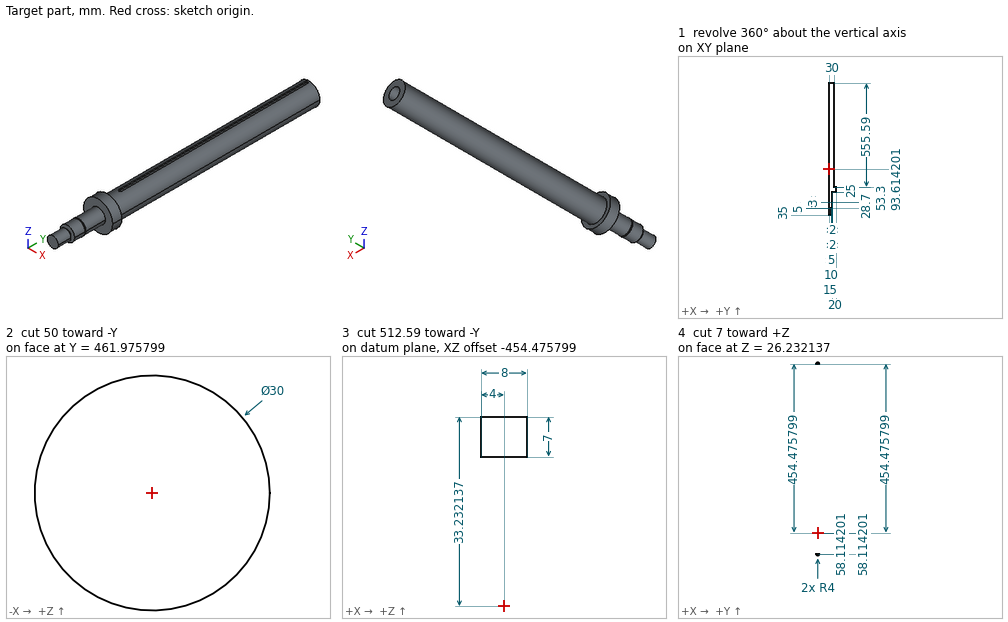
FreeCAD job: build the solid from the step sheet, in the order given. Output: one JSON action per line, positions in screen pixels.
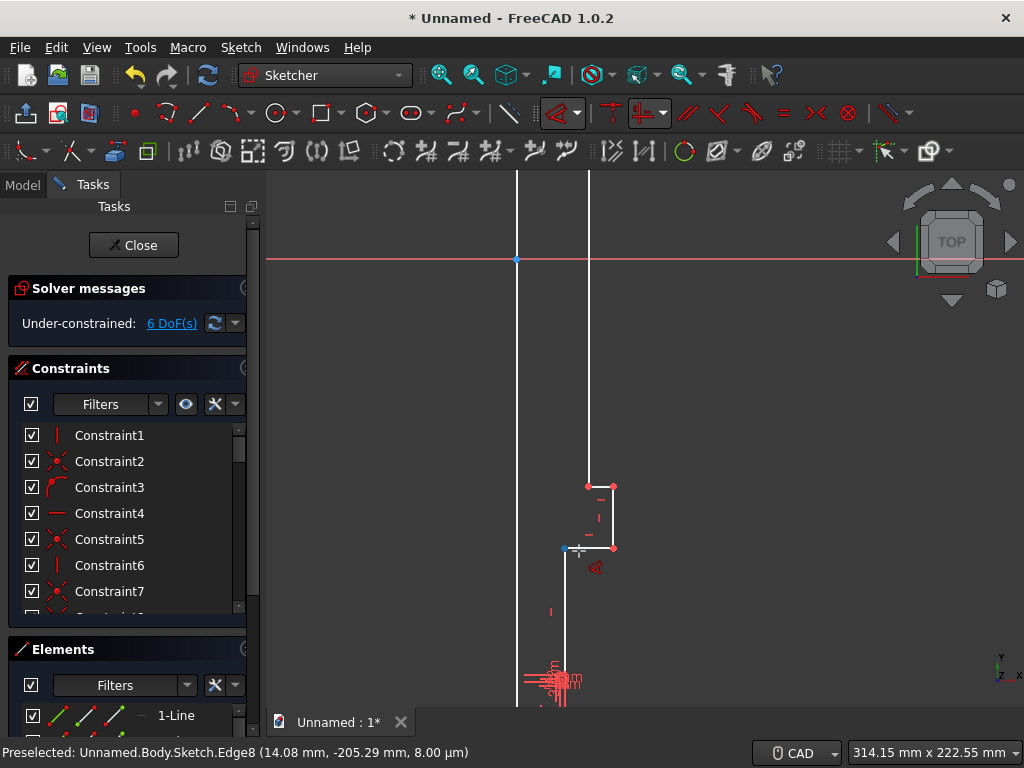
{"action": "left_click", "coordinate": [579, 548]}
{"action": "left_click", "coordinate": [589, 582]}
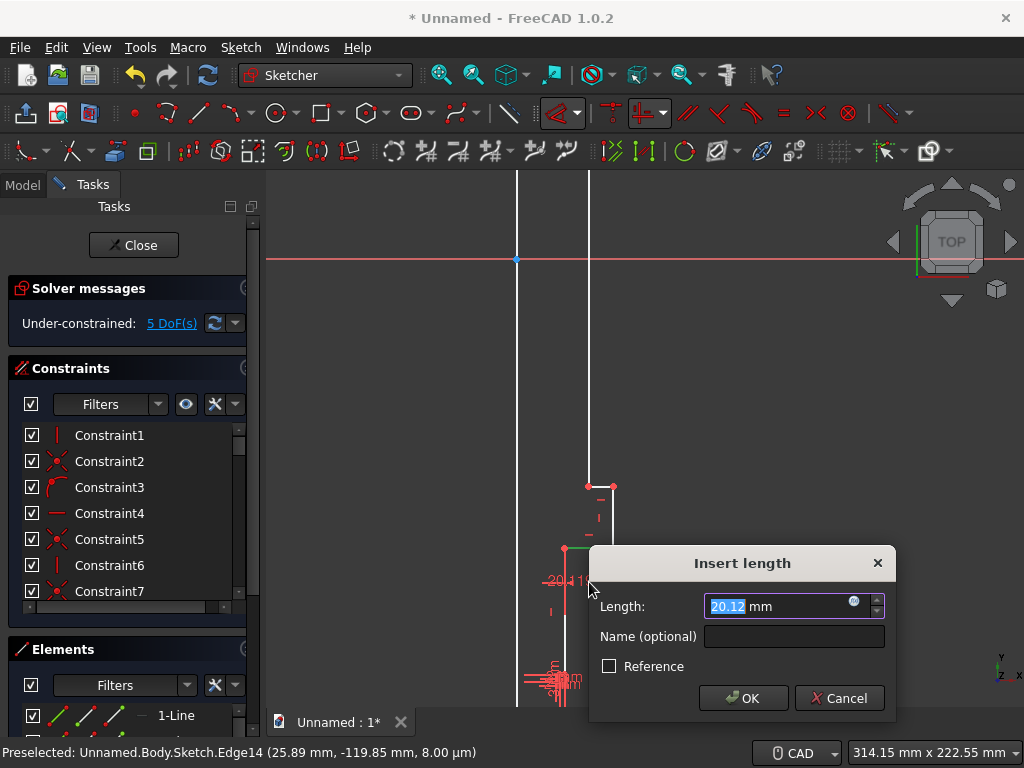
{"action": "type", "text": "20"}
{"action": "key", "text": "Return"}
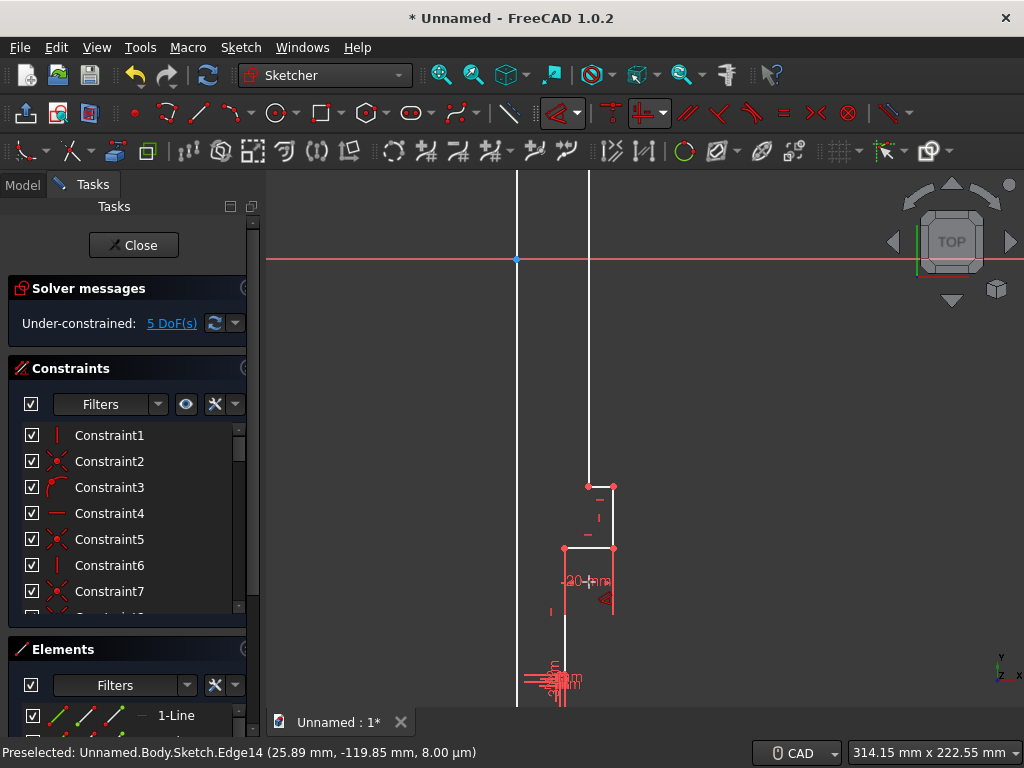
{"action": "left_click", "coordinate": [613, 530]}
{"action": "left_click", "coordinate": [647, 517]}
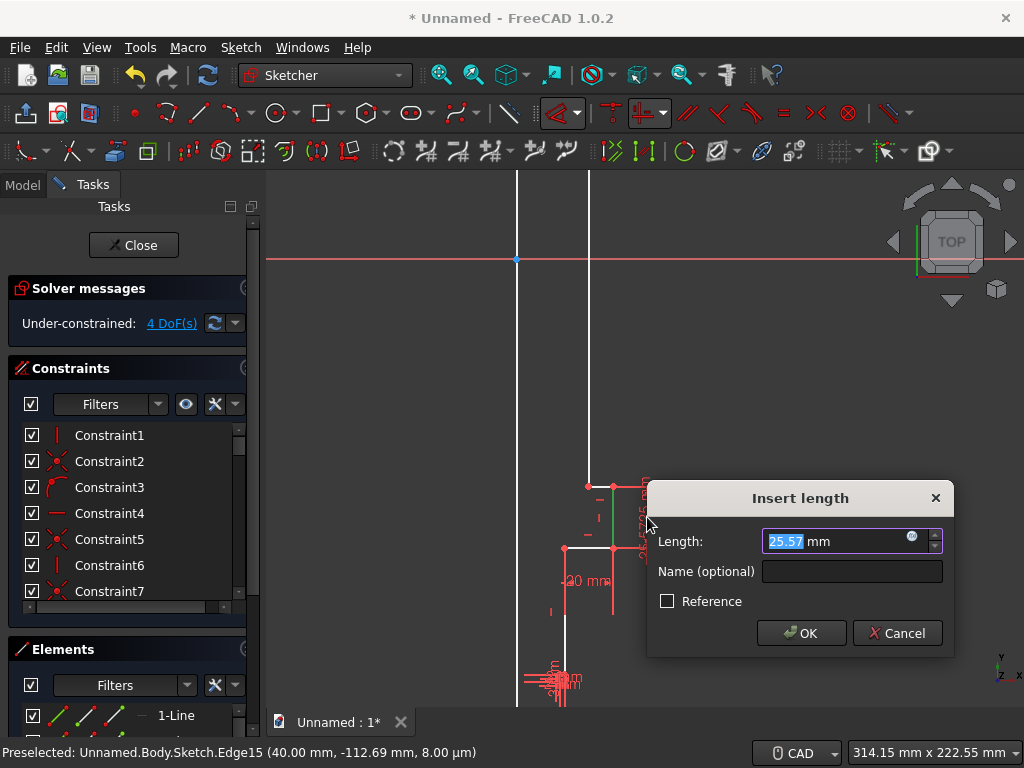
{"action": "type", "text": "25"}
{"action": "key", "text": "Return"}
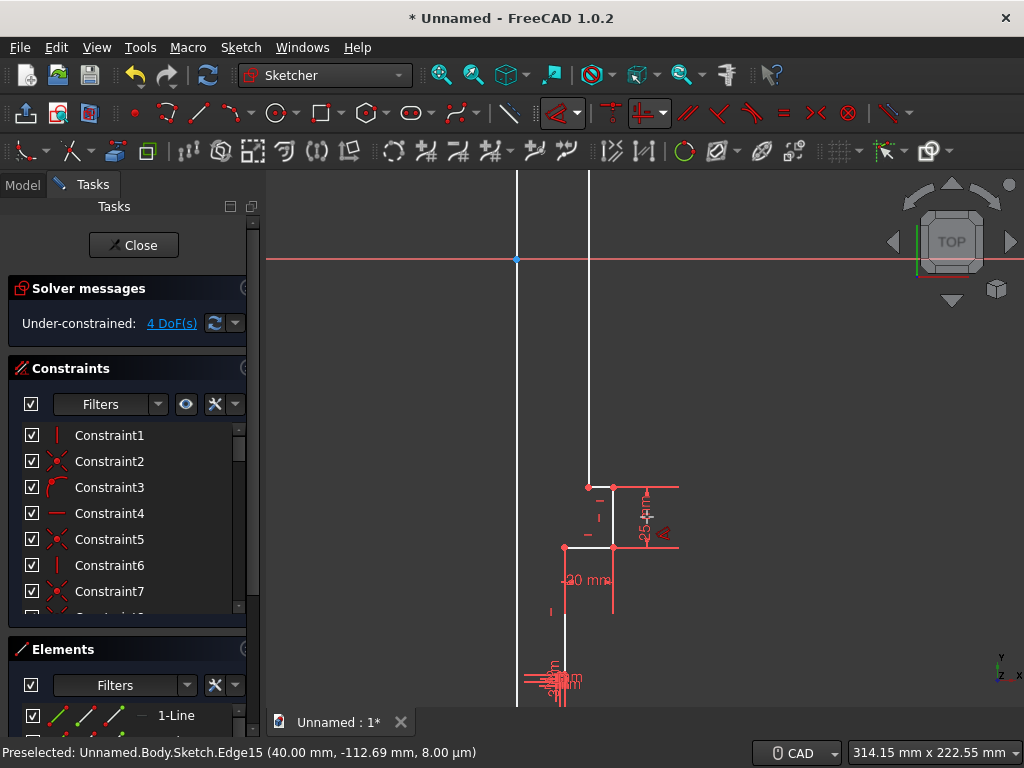
{"action": "scroll", "coordinate": [579, 551], "scroll_direction": "down", "scroll_amount": 8}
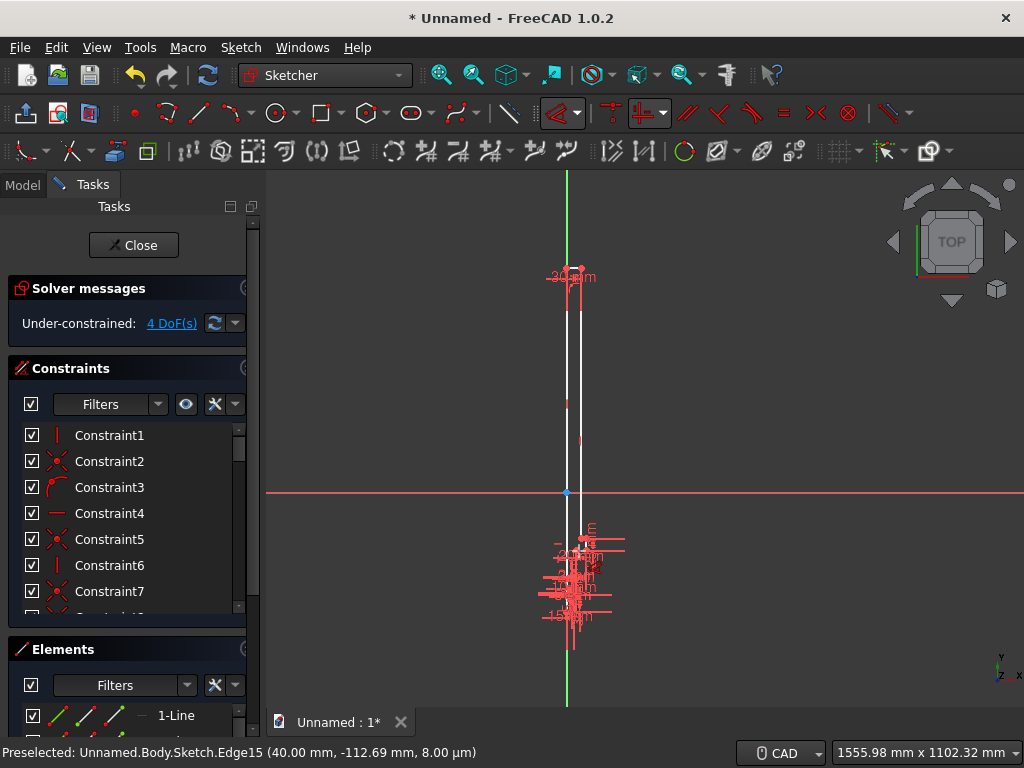
{"action": "scroll", "coordinate": [576, 588], "scroll_direction": "up", "scroll_amount": 6}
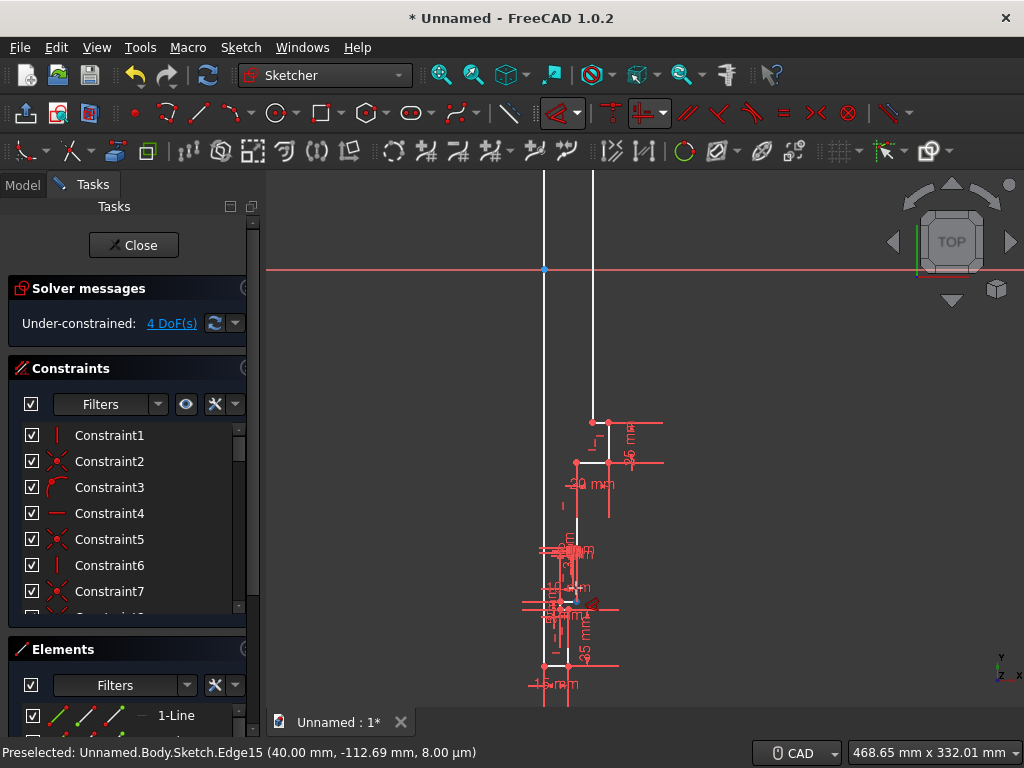
{"action": "left_click", "coordinate": [577, 587]}
{"action": "left_click", "coordinate": [659, 577]}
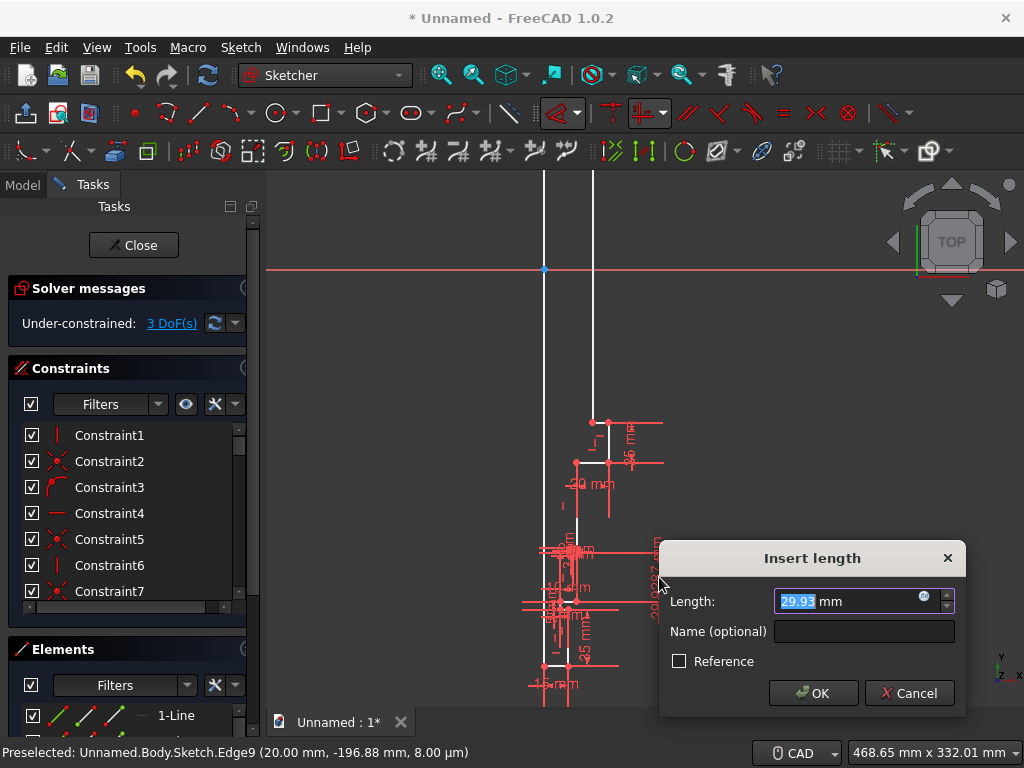
{"action": "type", "text": "28.7"}
{"action": "key", "text": "Return"}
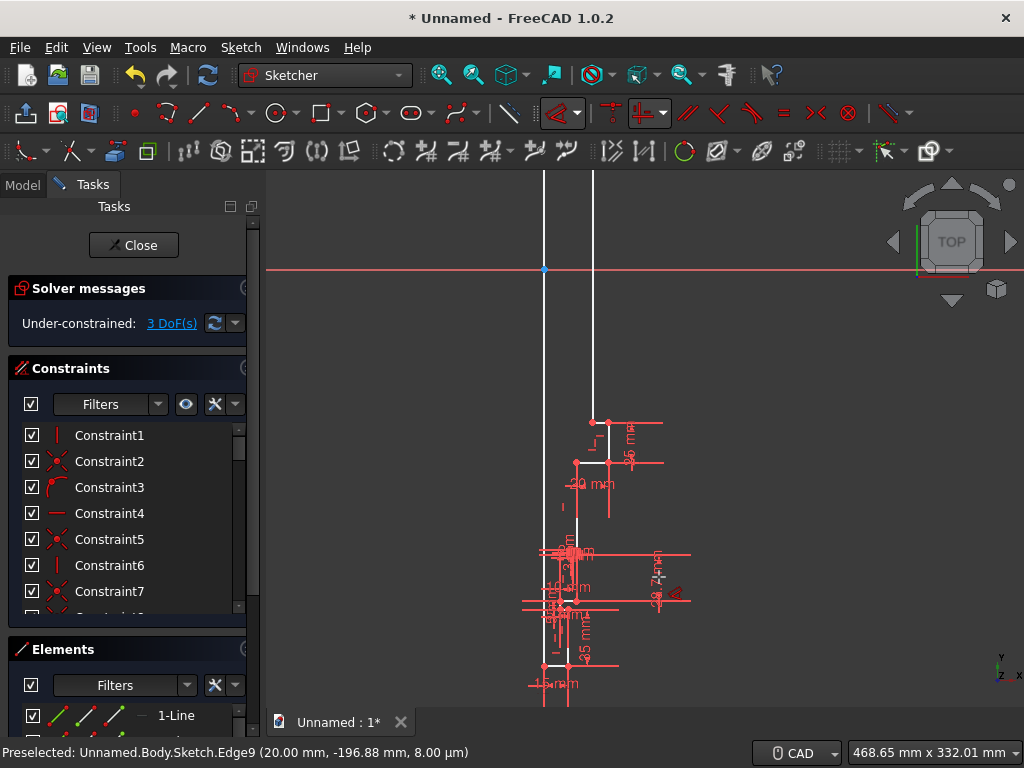
{"action": "left_click", "coordinate": [577, 524]}
{"action": "left_click", "coordinate": [611, 507]}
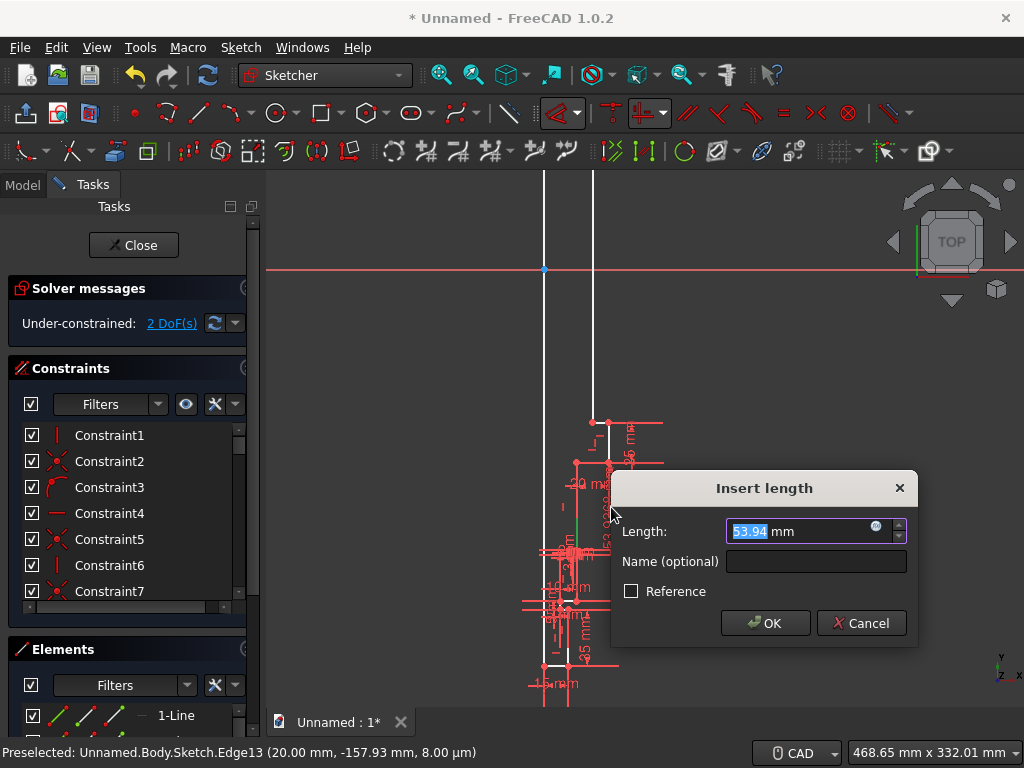
{"action": "type", "text": "53.3"}
{"action": "key", "text": "Return"}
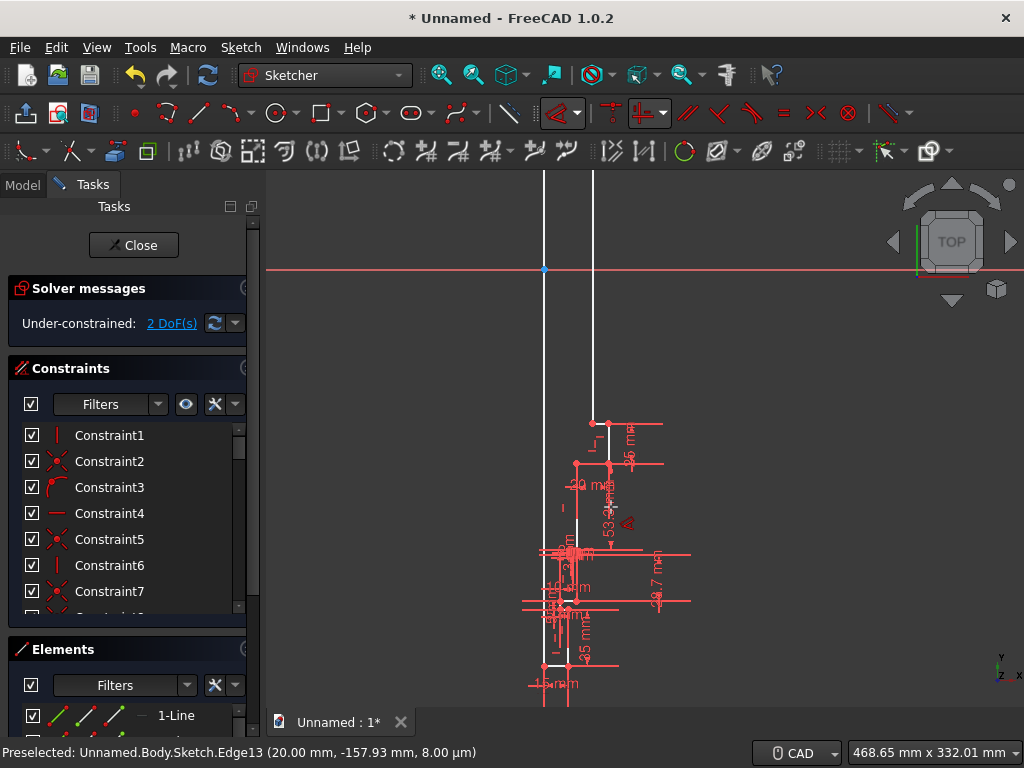
{"action": "left_click", "coordinate": [593, 244]}
{"action": "left_click", "coordinate": [627, 311]}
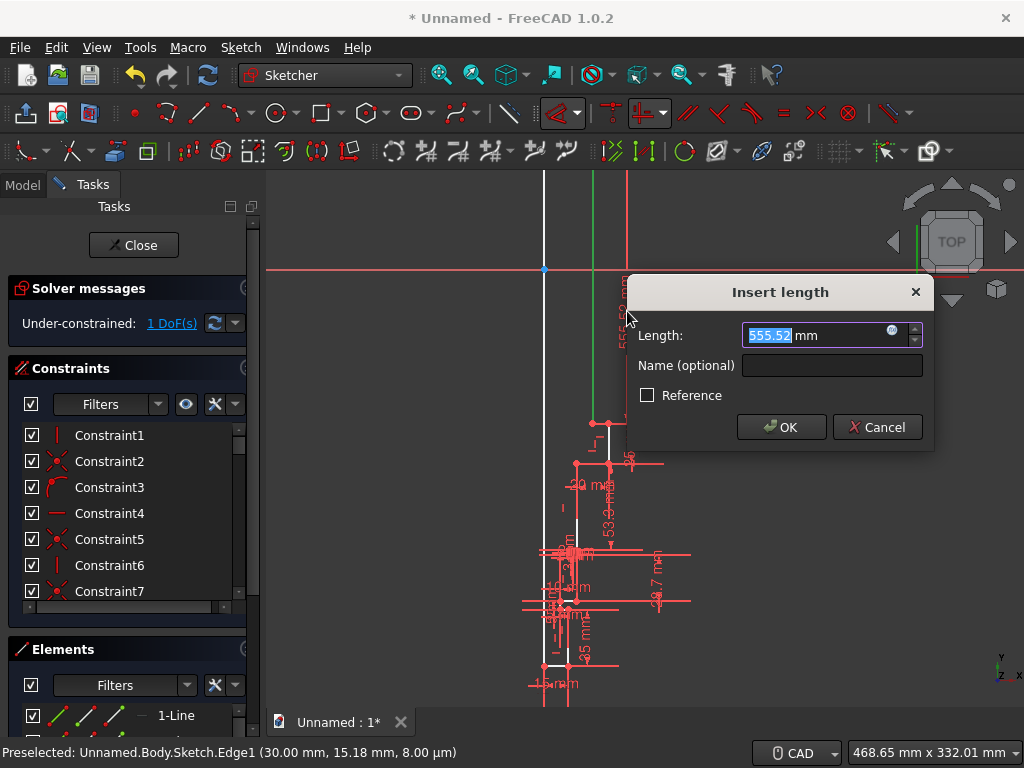
{"action": "type", "text": "555.59"}
{"action": "key", "text": "Return"}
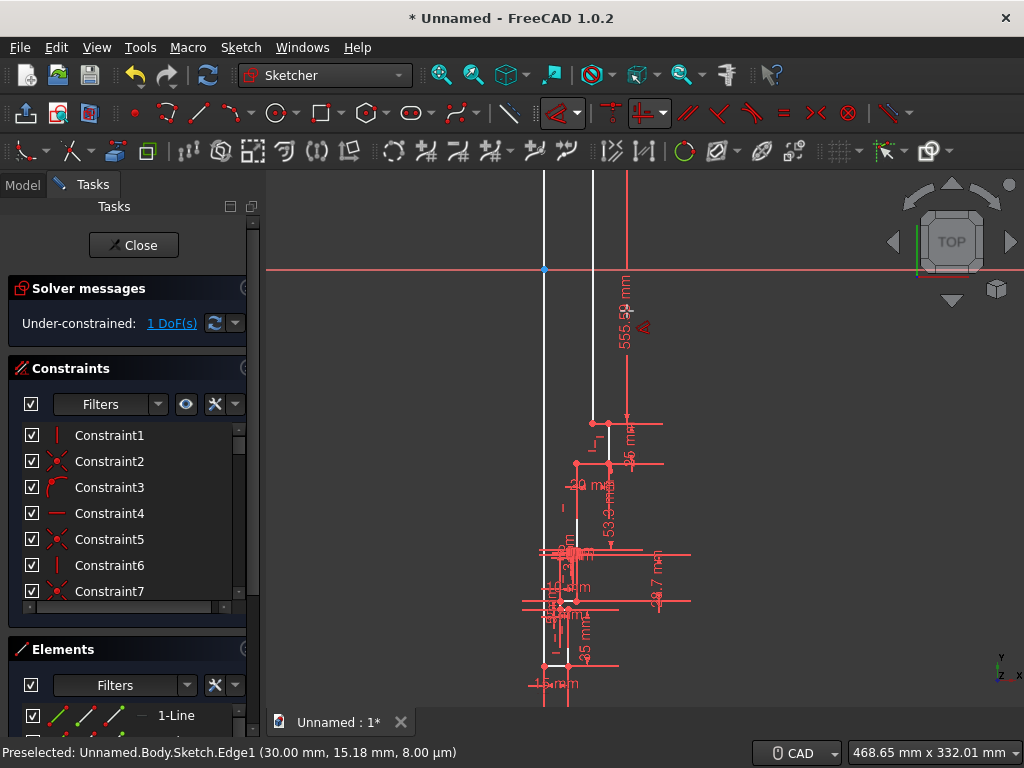
{"action": "left_click", "coordinate": [593, 424]}
{"action": "left_click", "coordinate": [510, 347]}